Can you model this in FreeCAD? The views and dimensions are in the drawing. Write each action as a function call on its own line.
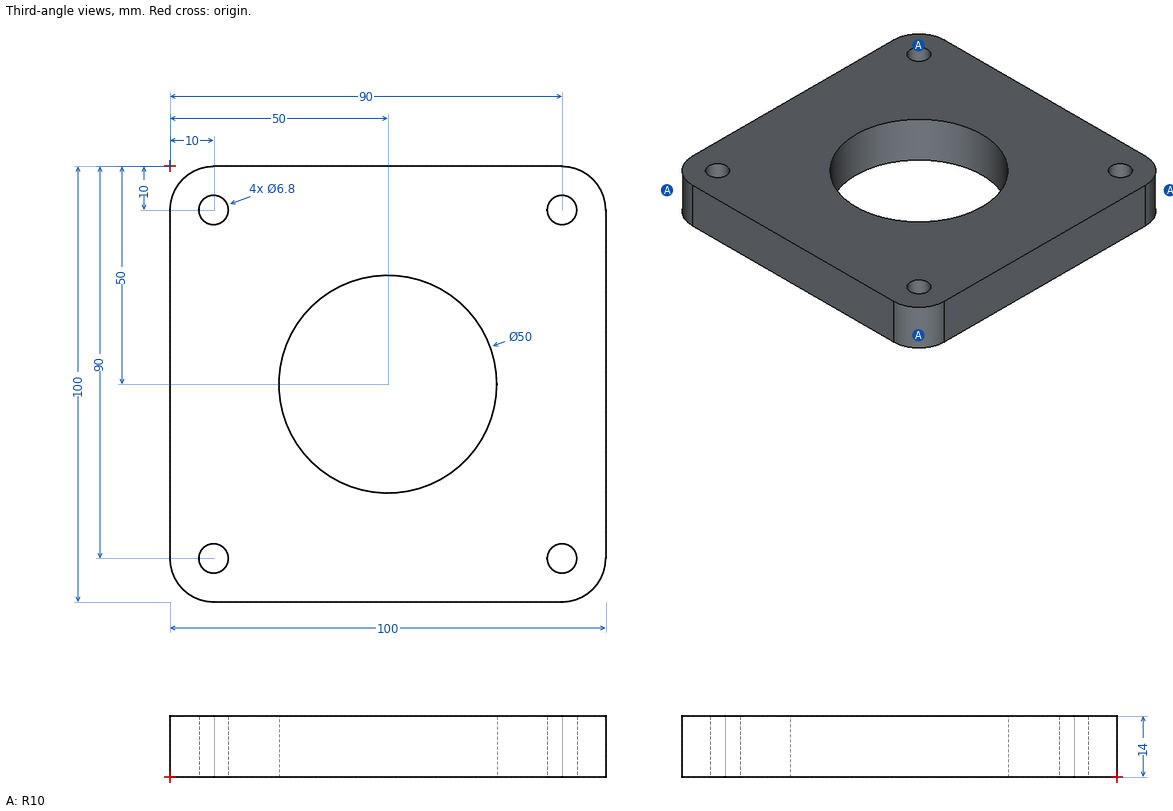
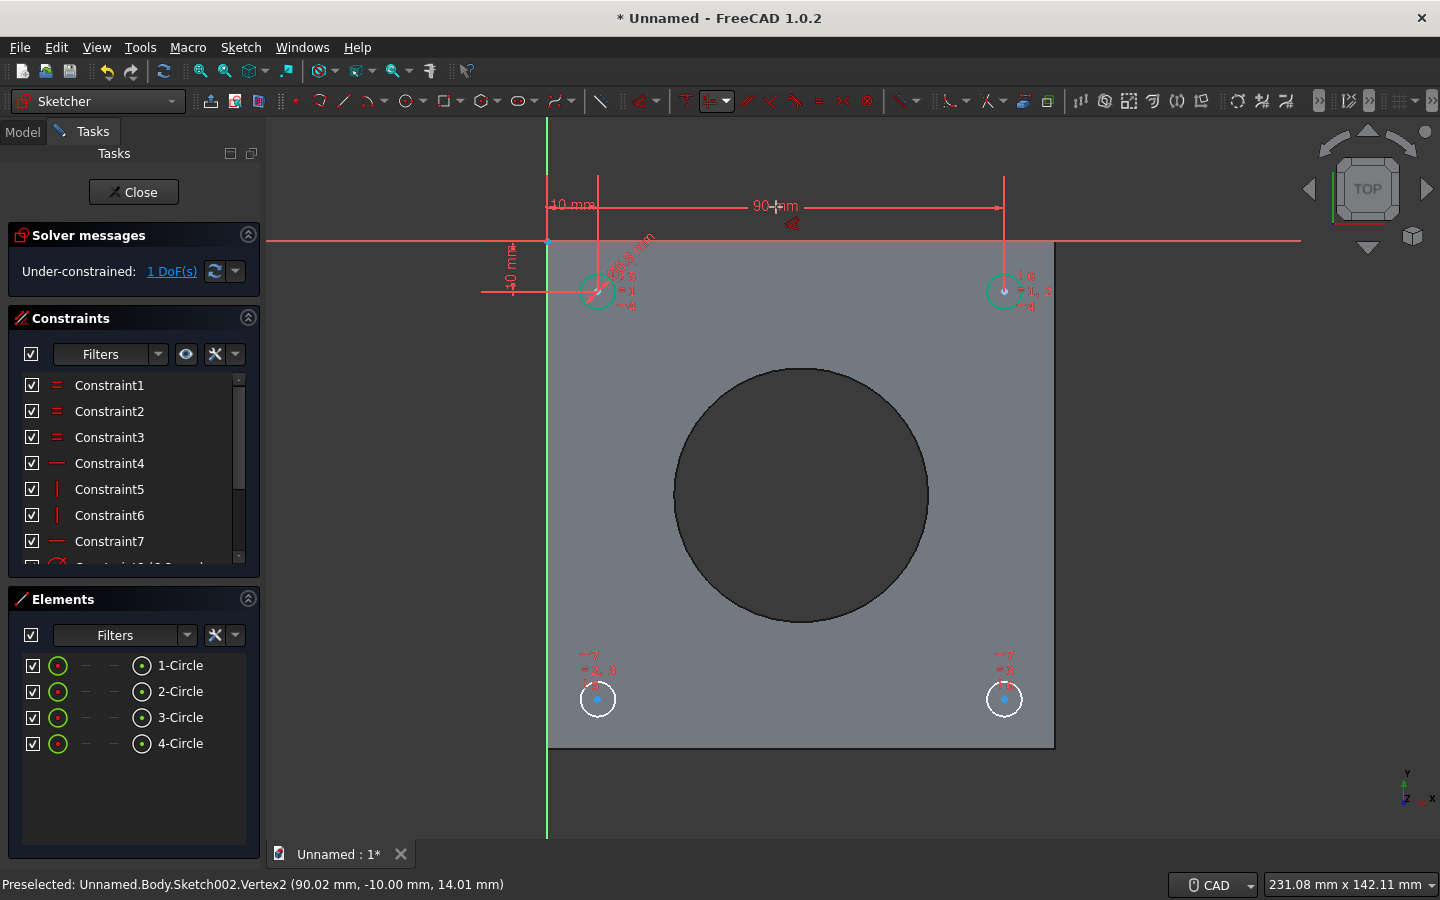
click(598, 699)
click(513, 470)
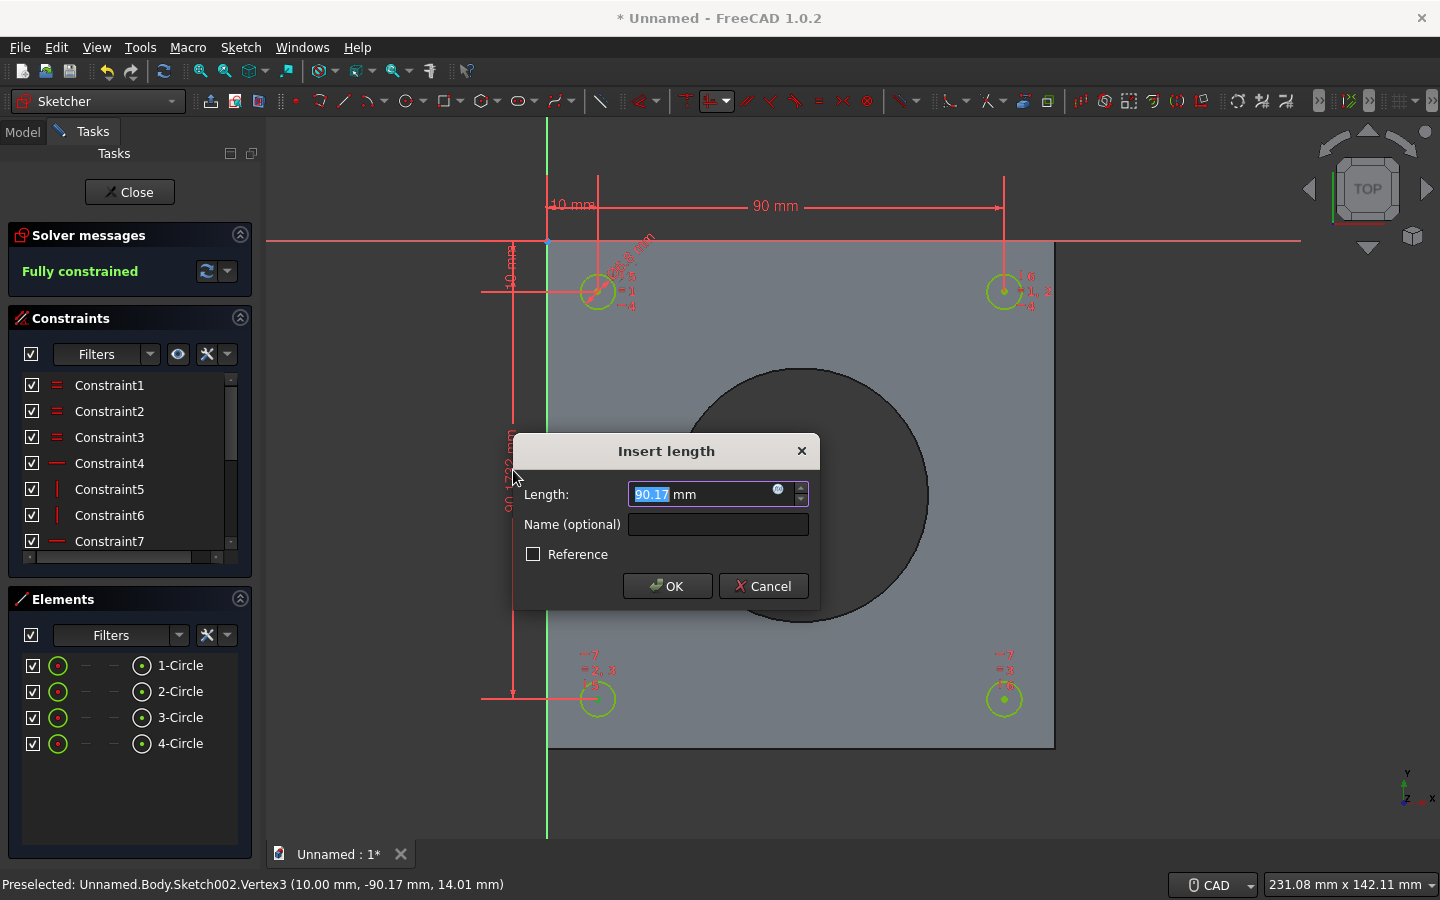
text(90)
key(Return)
key(Escape)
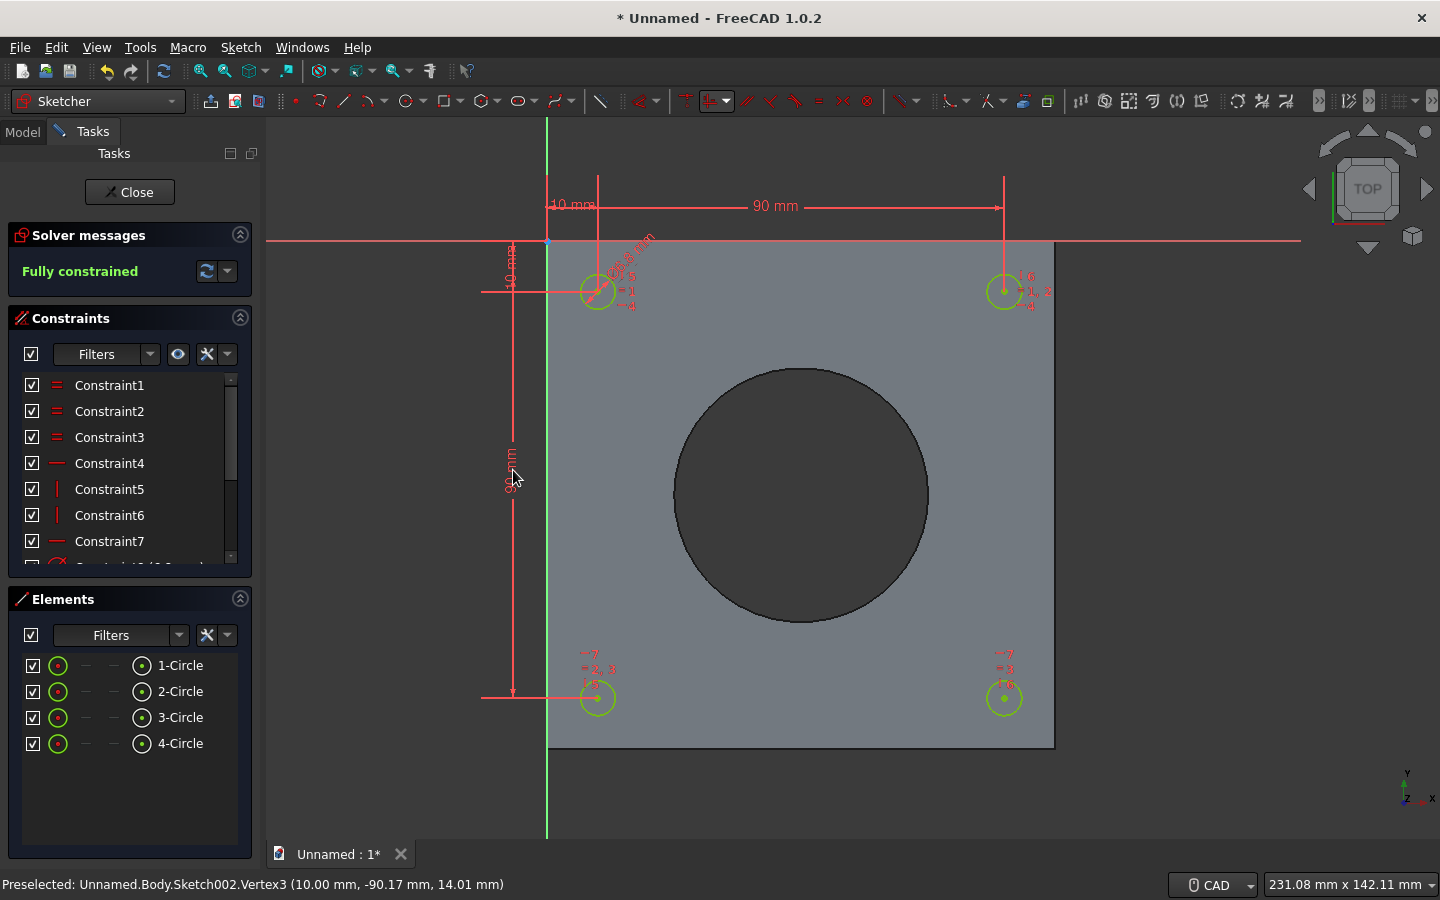
click(130, 192)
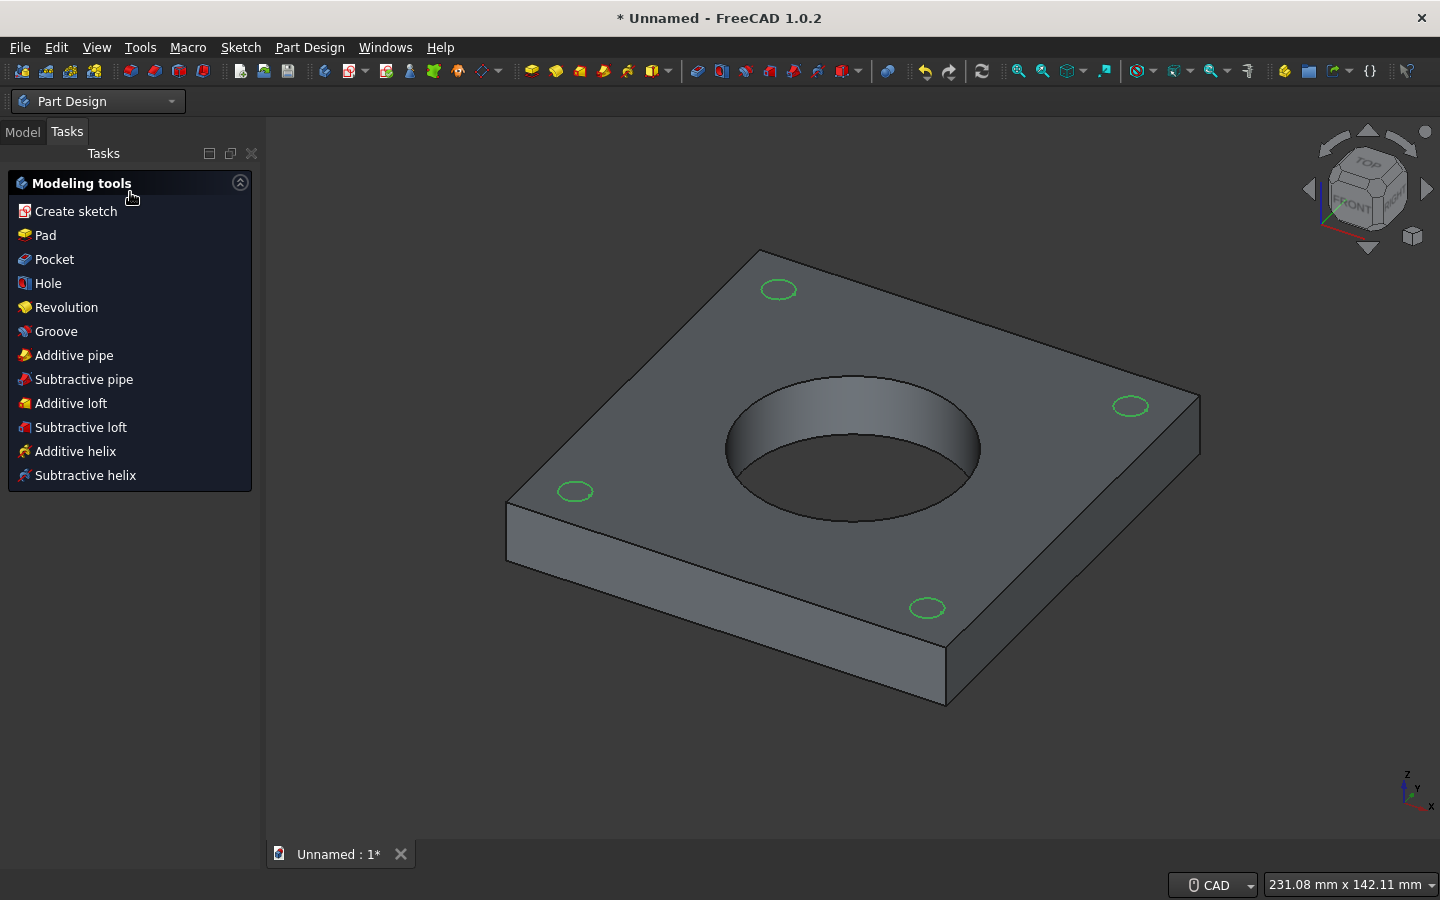
click(698, 72)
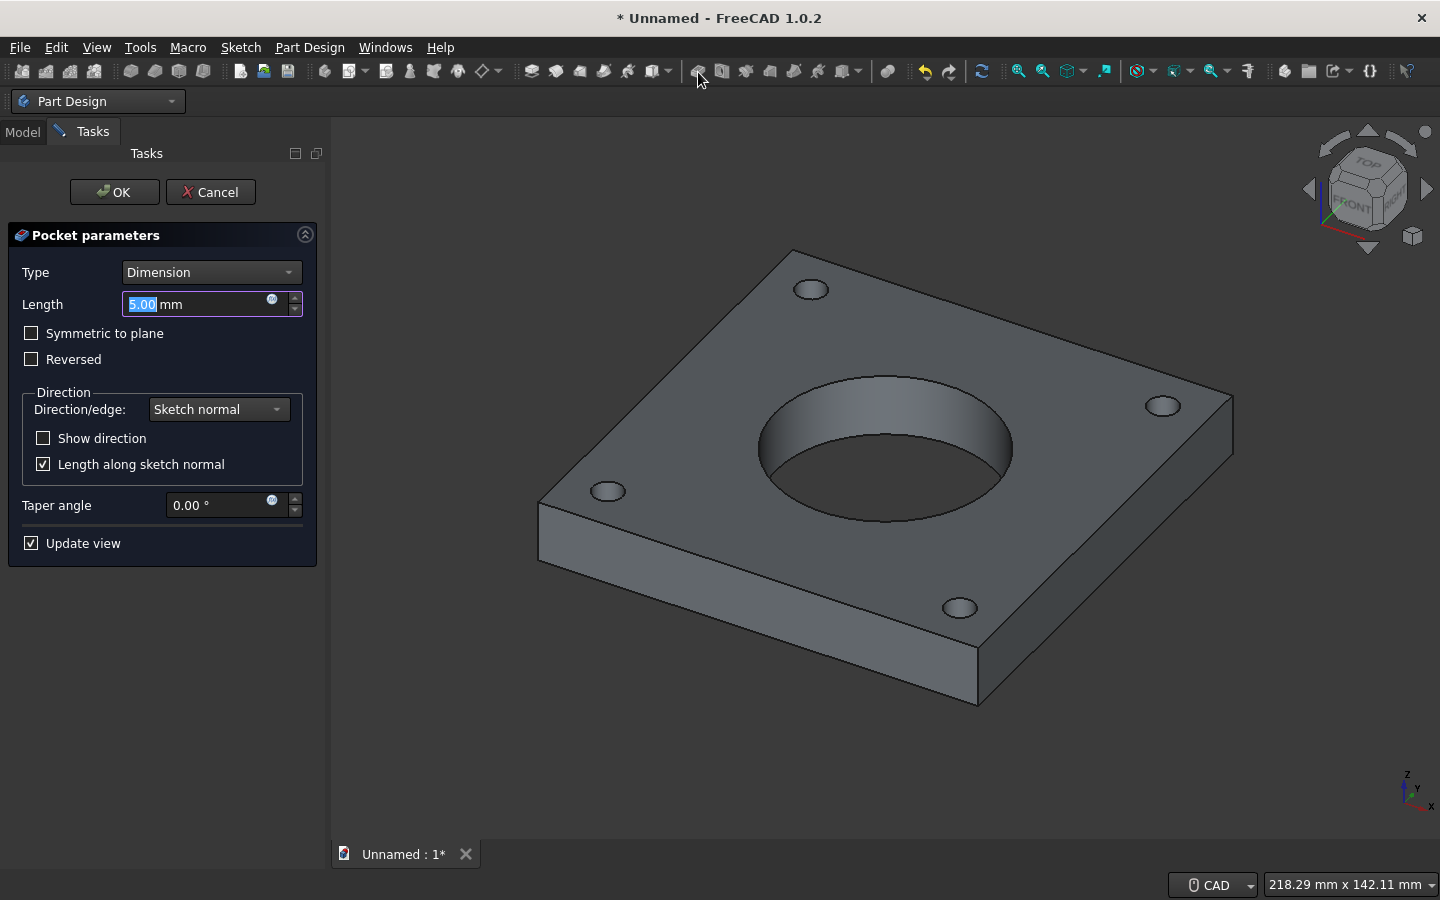
click(212, 272)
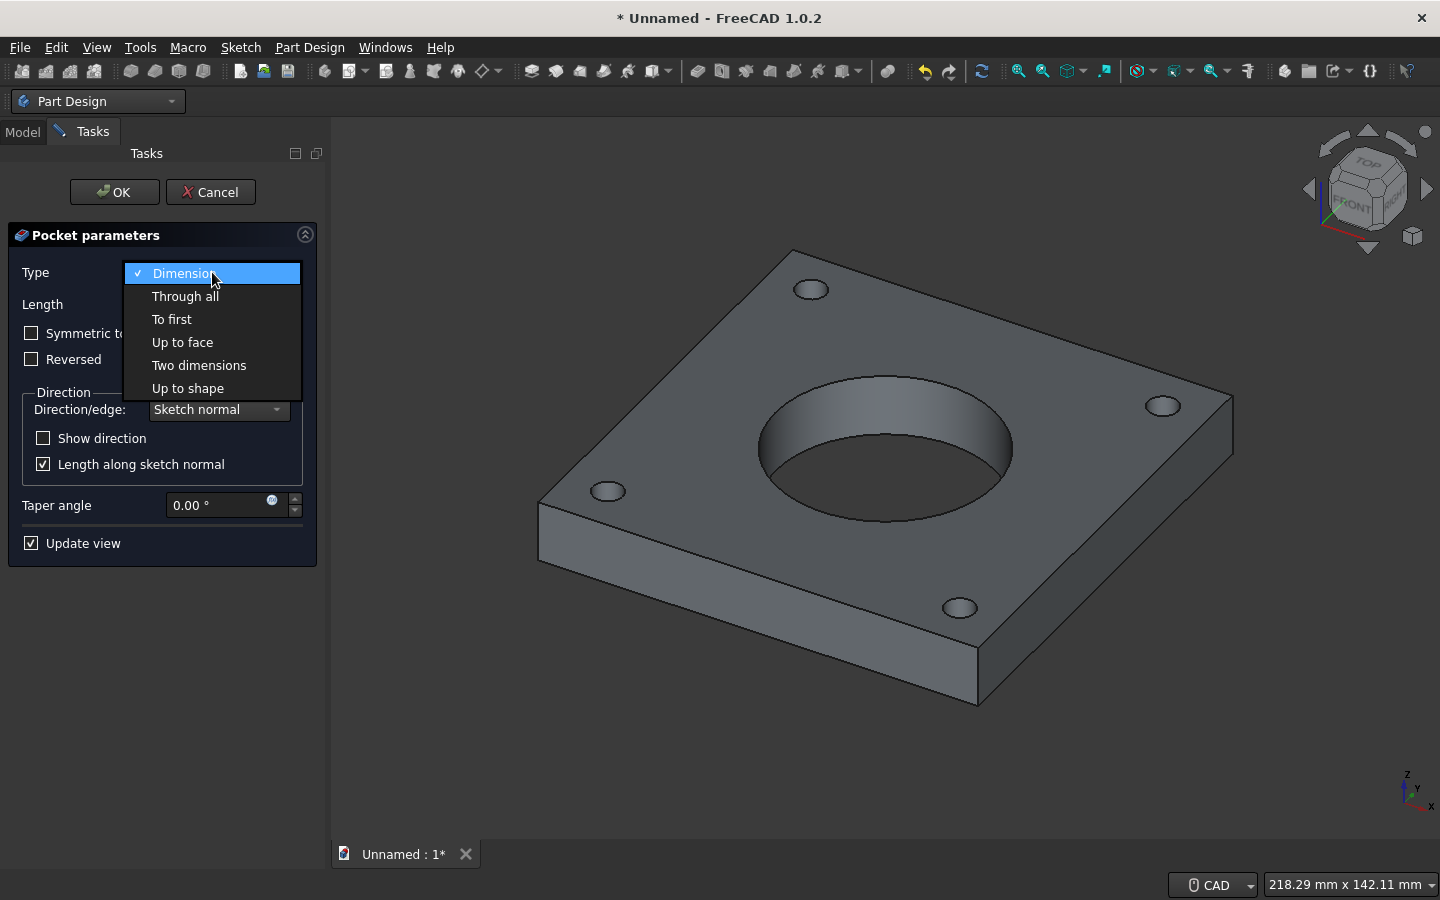
click(212, 296)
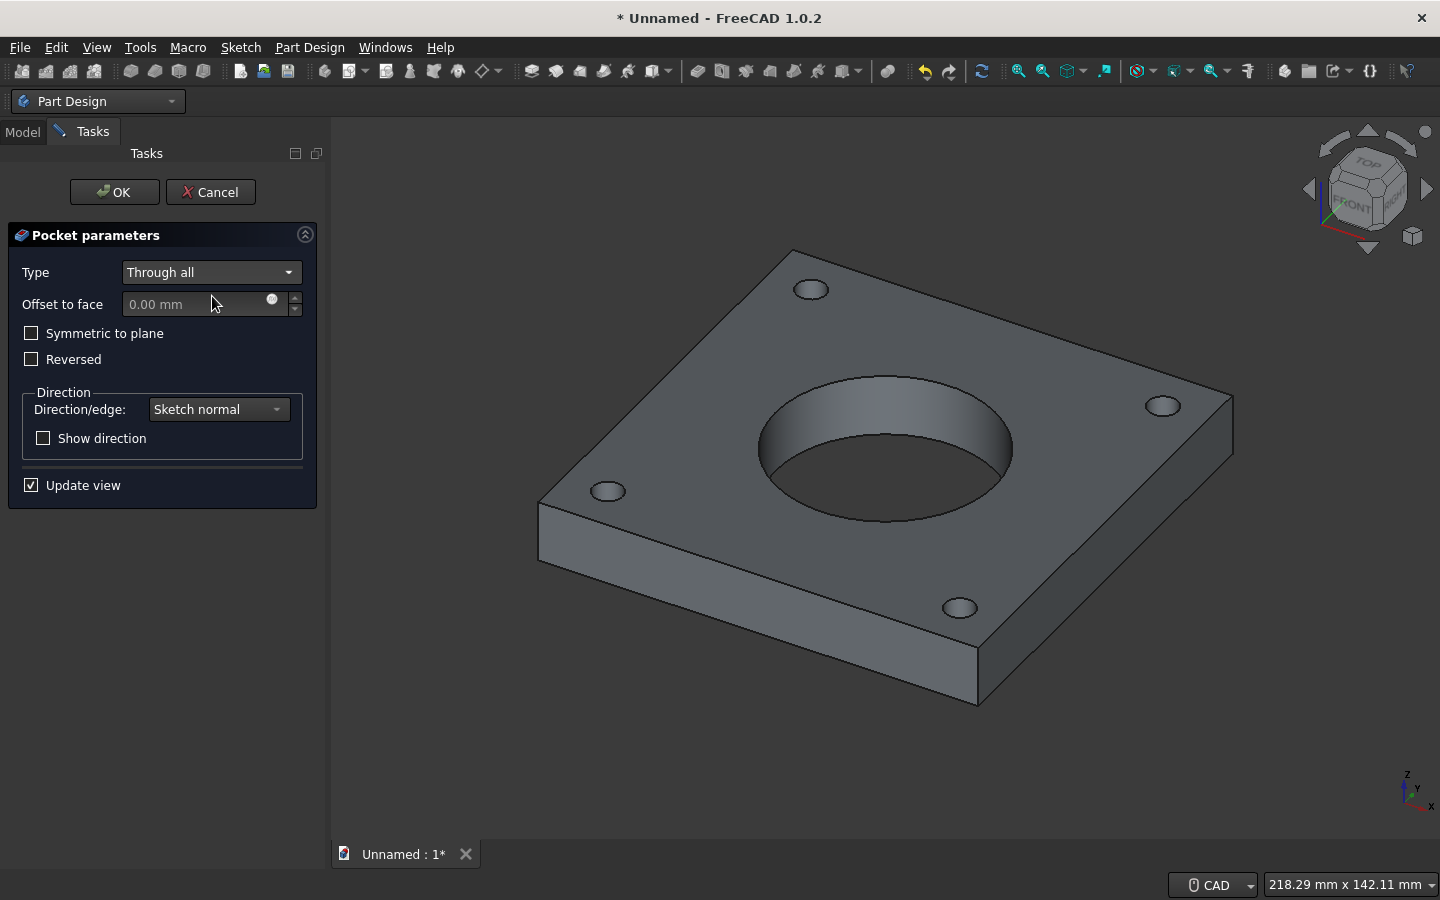
click(115, 192)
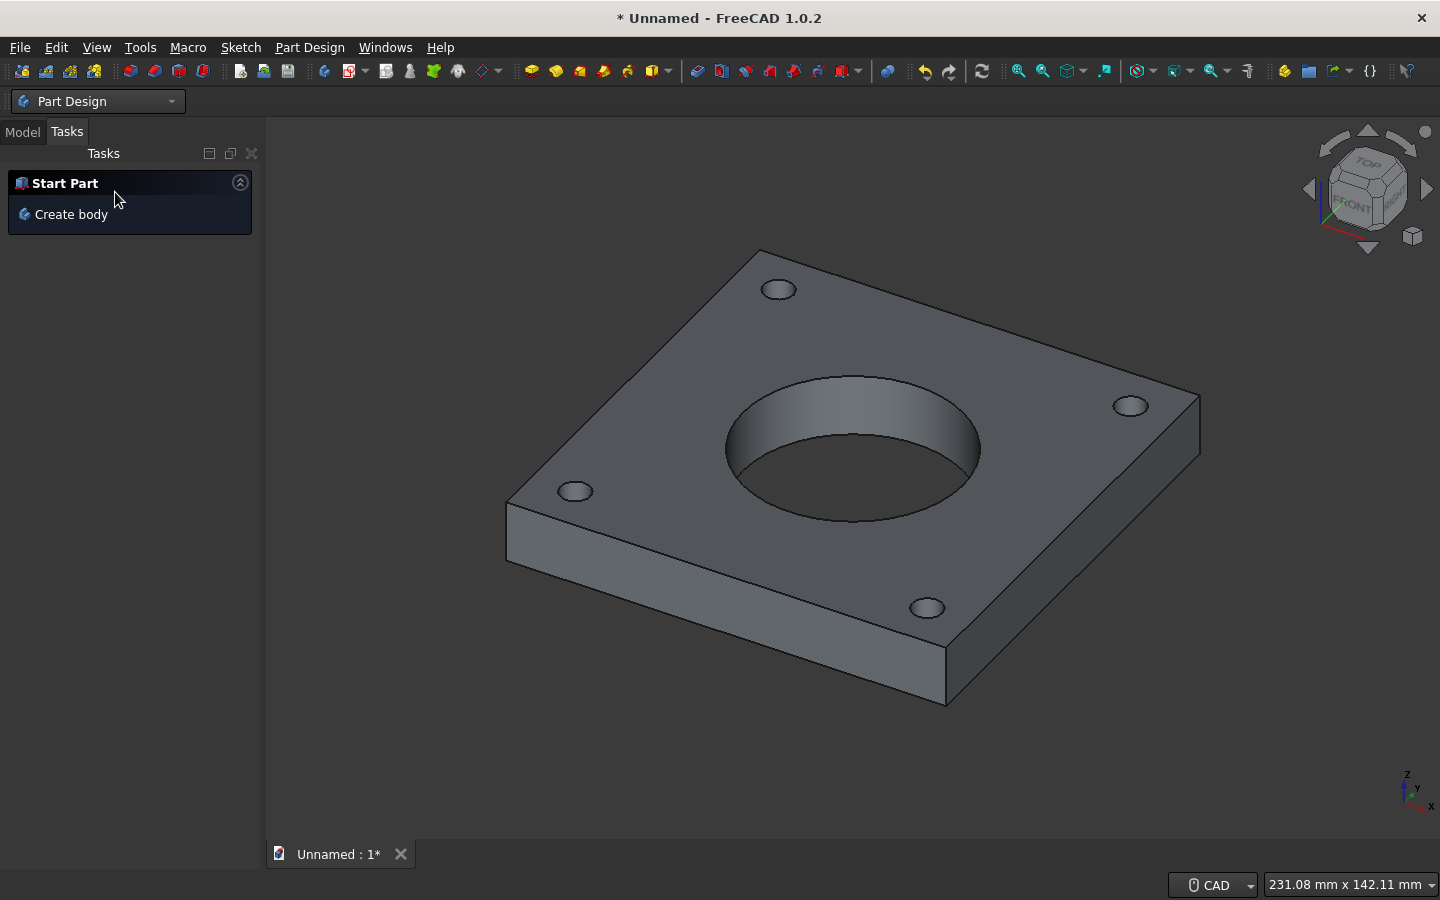
click(946, 676)